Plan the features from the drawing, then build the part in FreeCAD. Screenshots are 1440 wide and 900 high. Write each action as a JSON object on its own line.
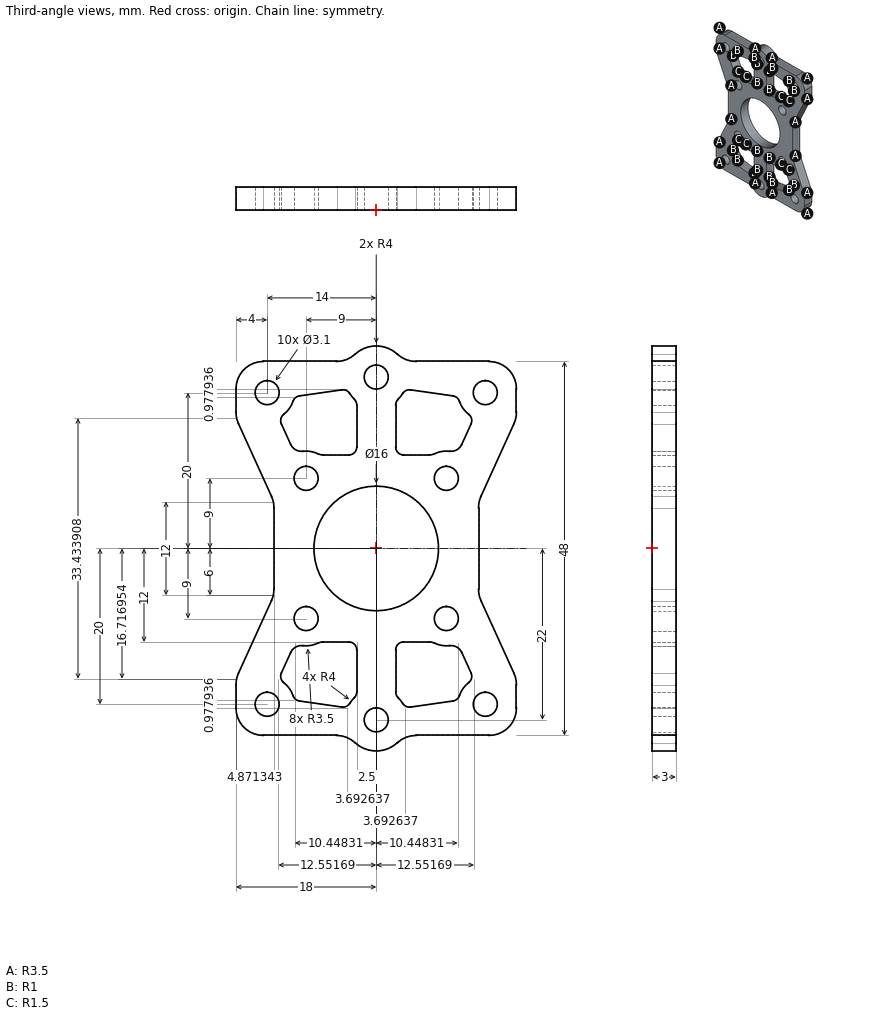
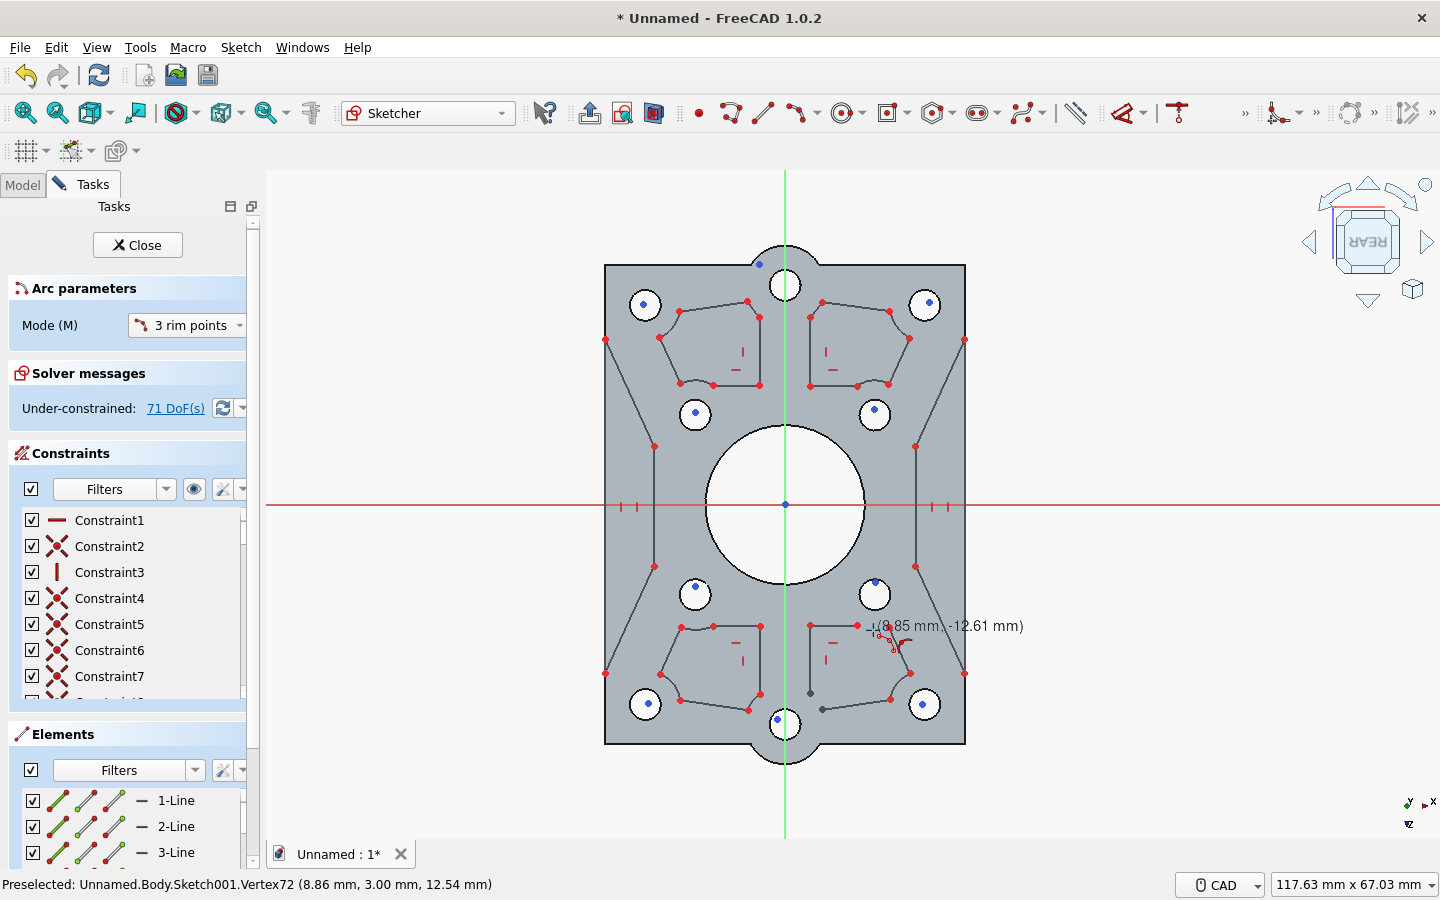
{"action": "left_click", "coordinate": [810, 694]}
{"action": "left_click", "coordinate": [822, 710]}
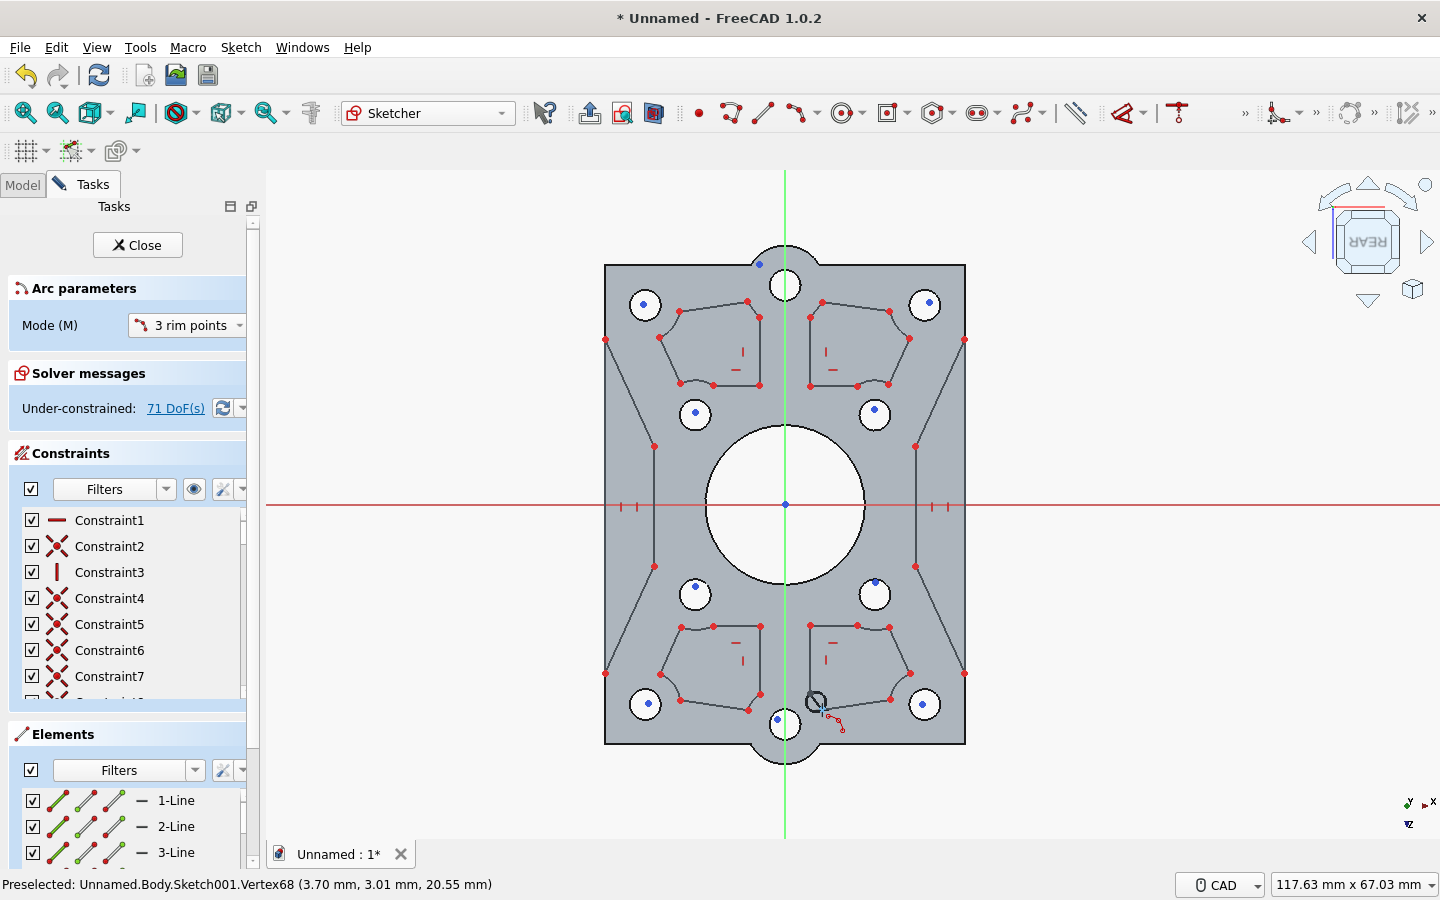
{"action": "scroll", "coordinate": [817, 700], "scroll_direction": "up", "scroll_amount": 13}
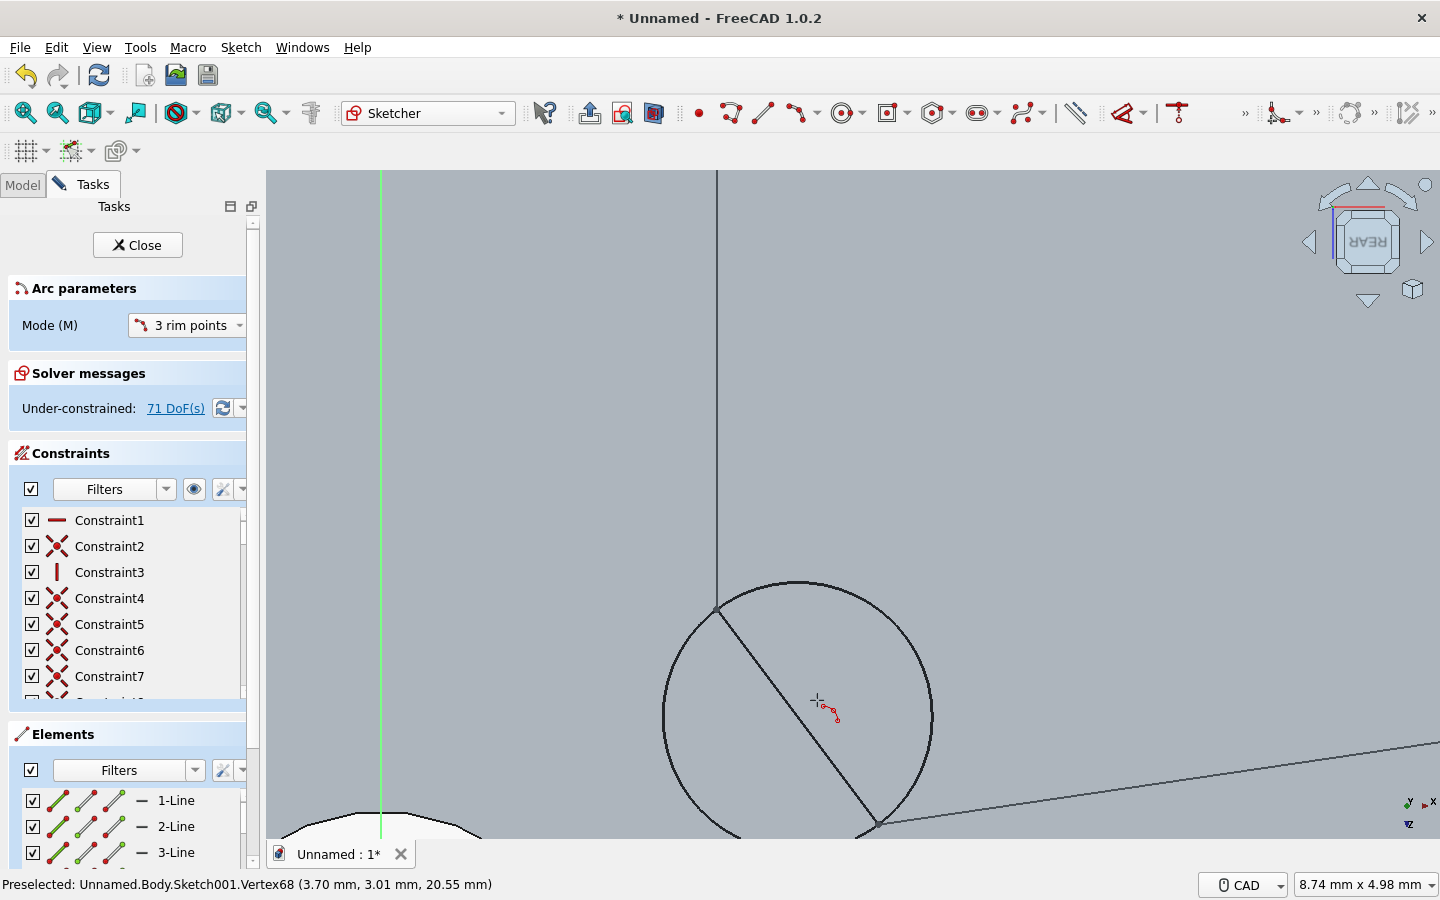
{"action": "left_click", "coordinate": [811, 697]}
{"action": "key", "text": "Escape"}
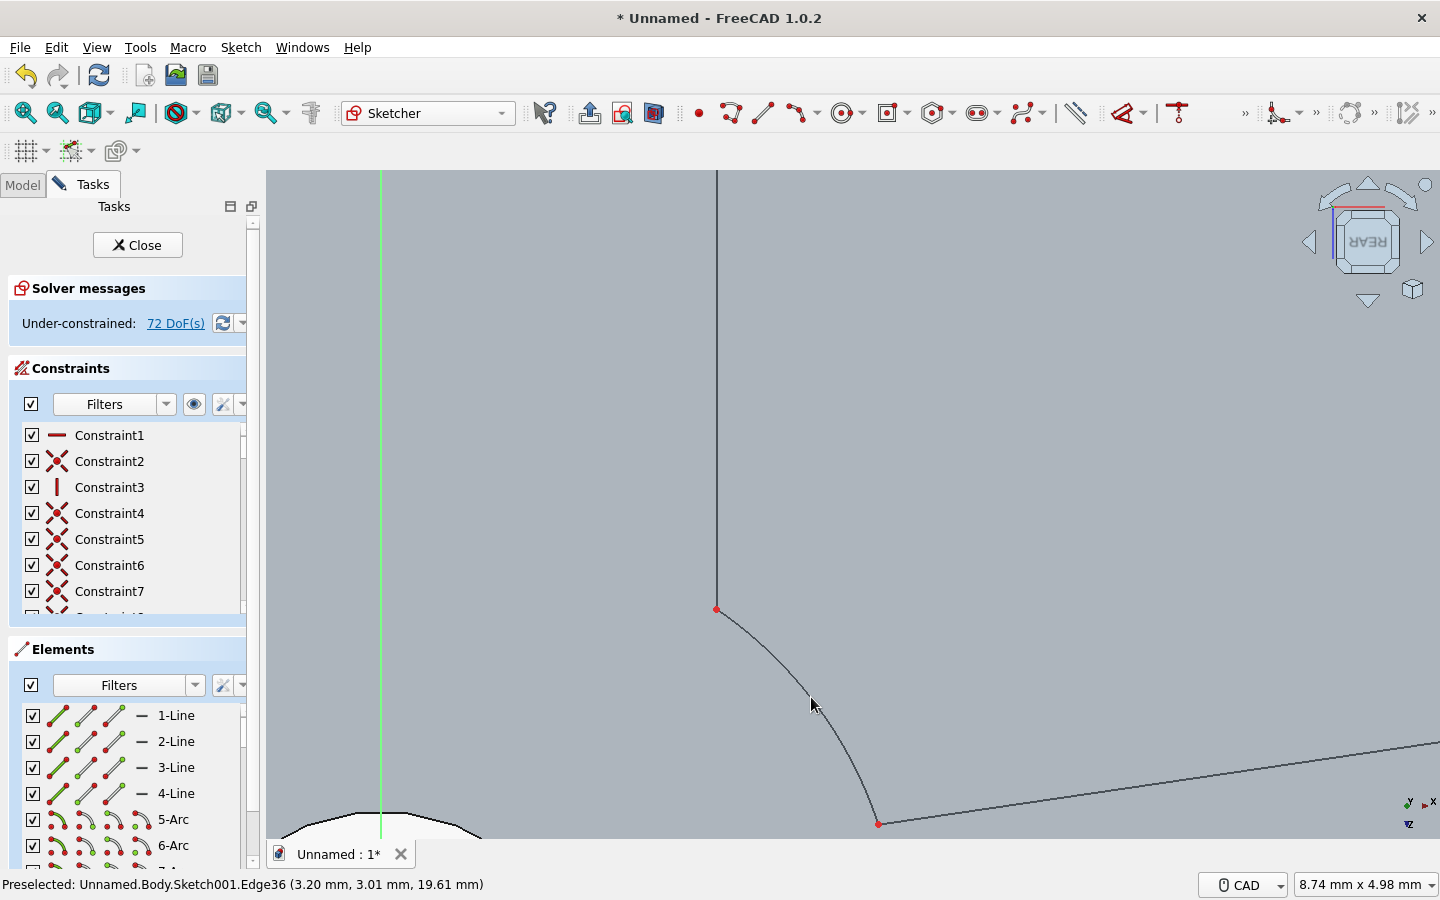
{"action": "scroll", "coordinate": [817, 700], "scroll_direction": "down", "scroll_amount": 13}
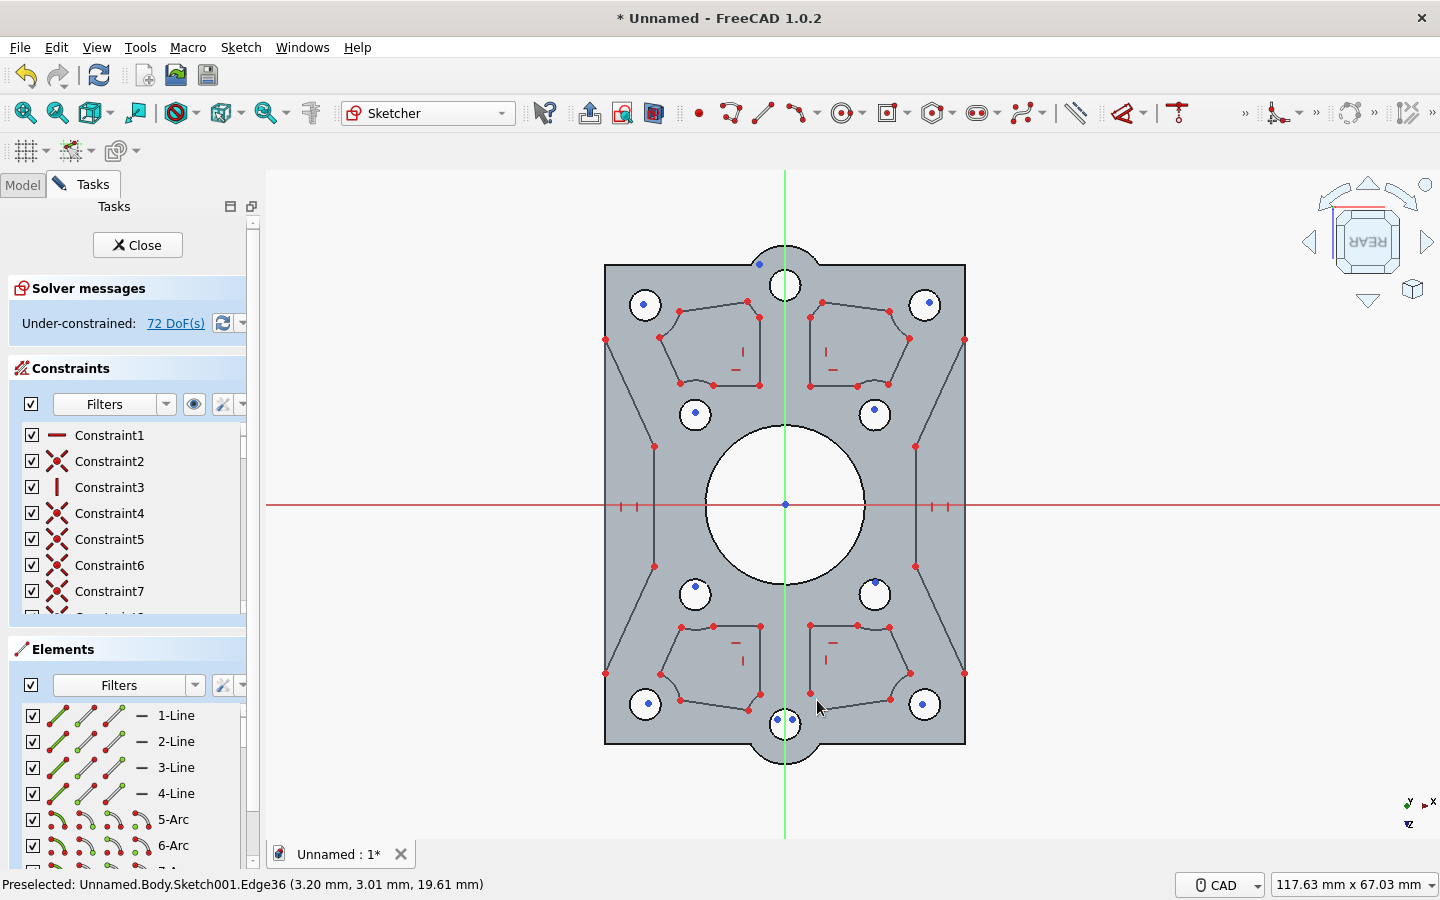
{"action": "scroll", "coordinate": [751, 307], "scroll_direction": "up", "scroll_amount": 5}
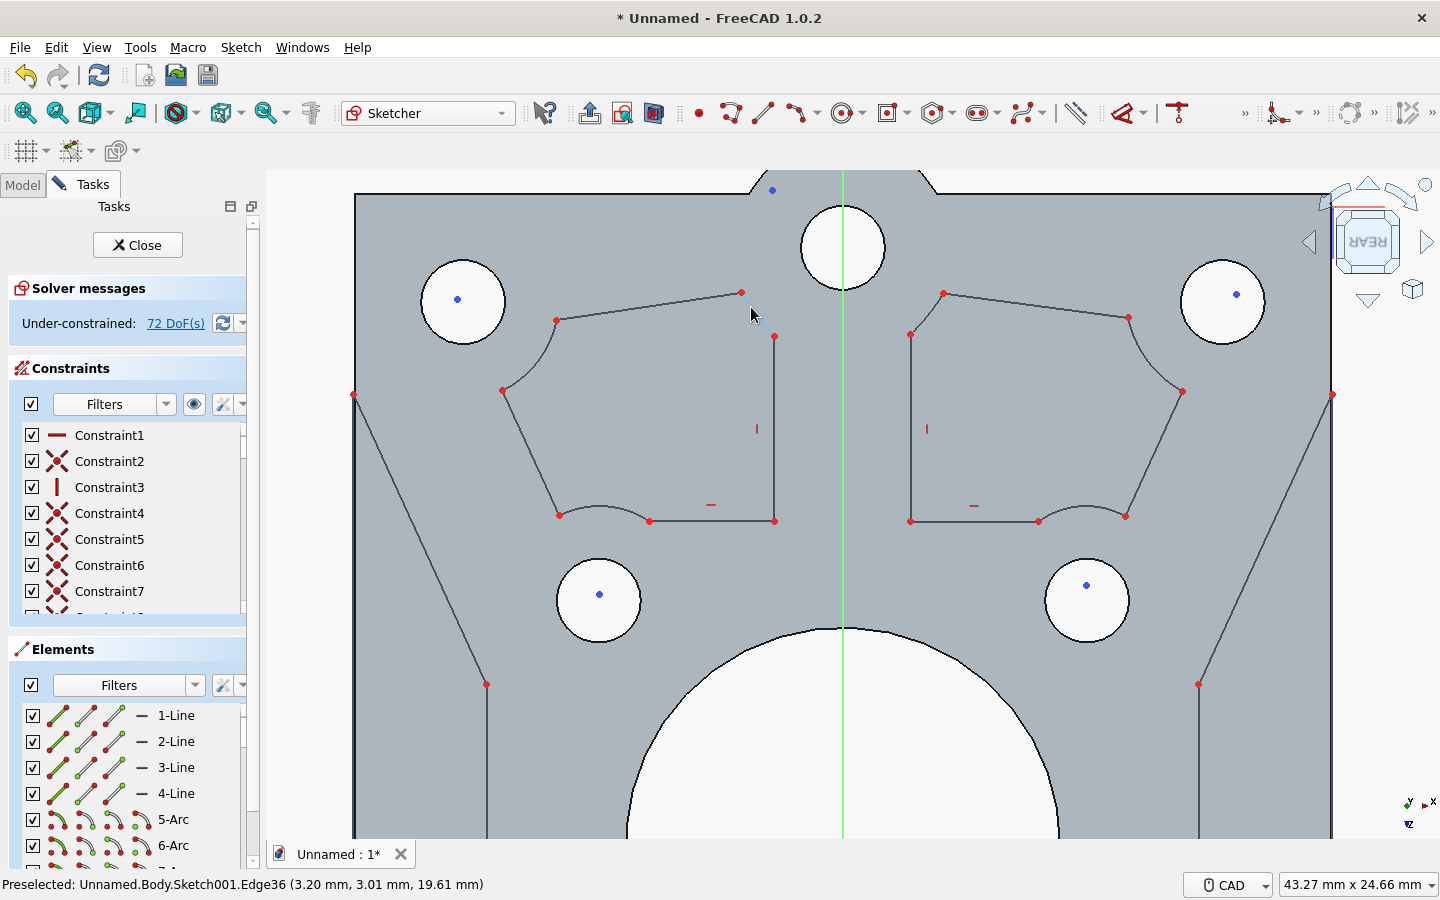
{"action": "left_click", "coordinate": [751, 306]}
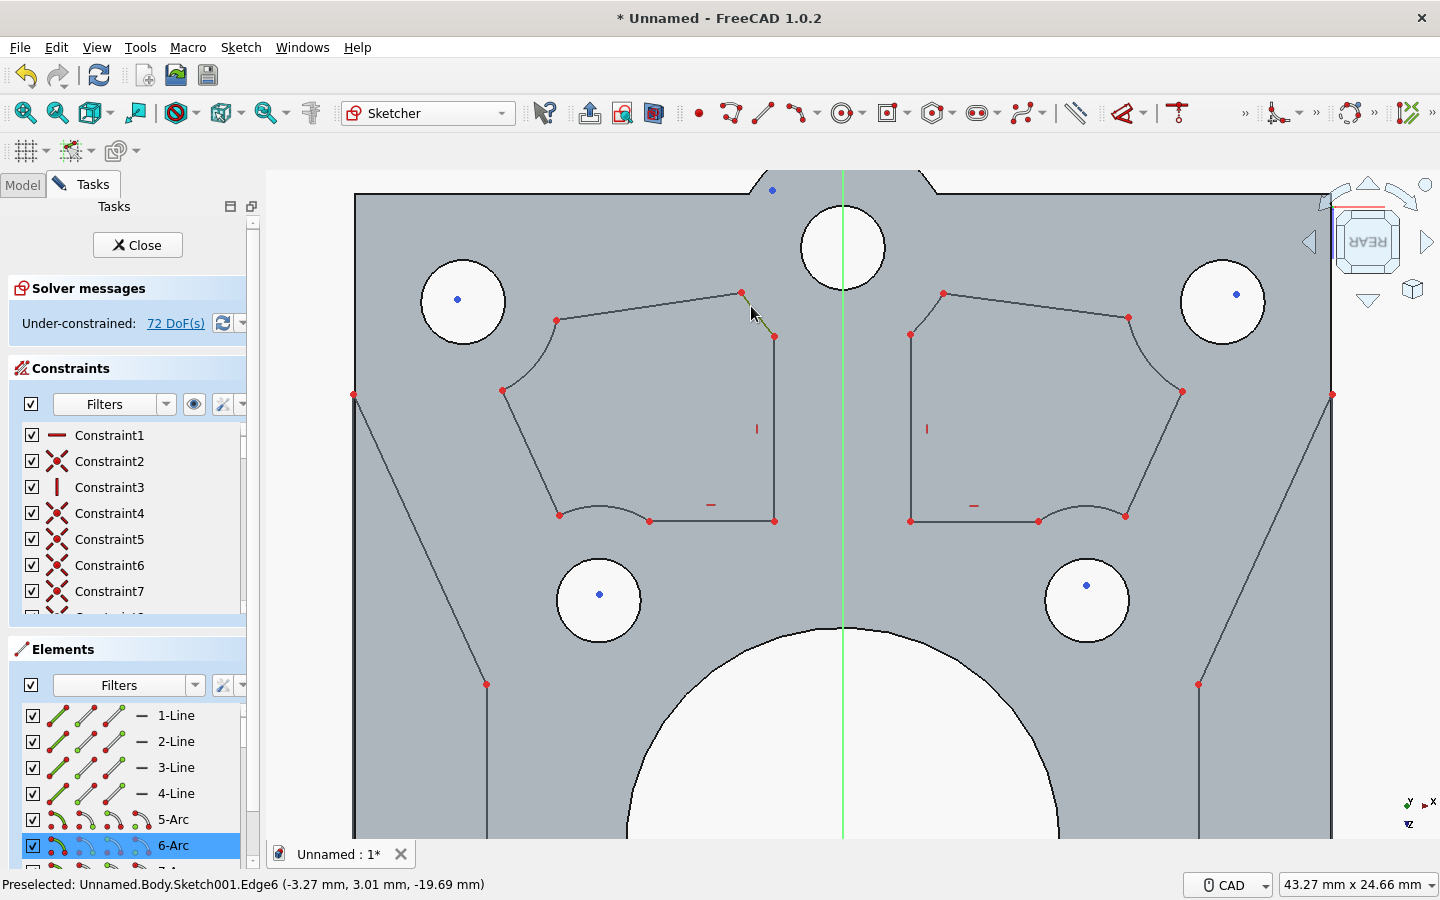
{"action": "left_click", "coordinate": [922, 323]}